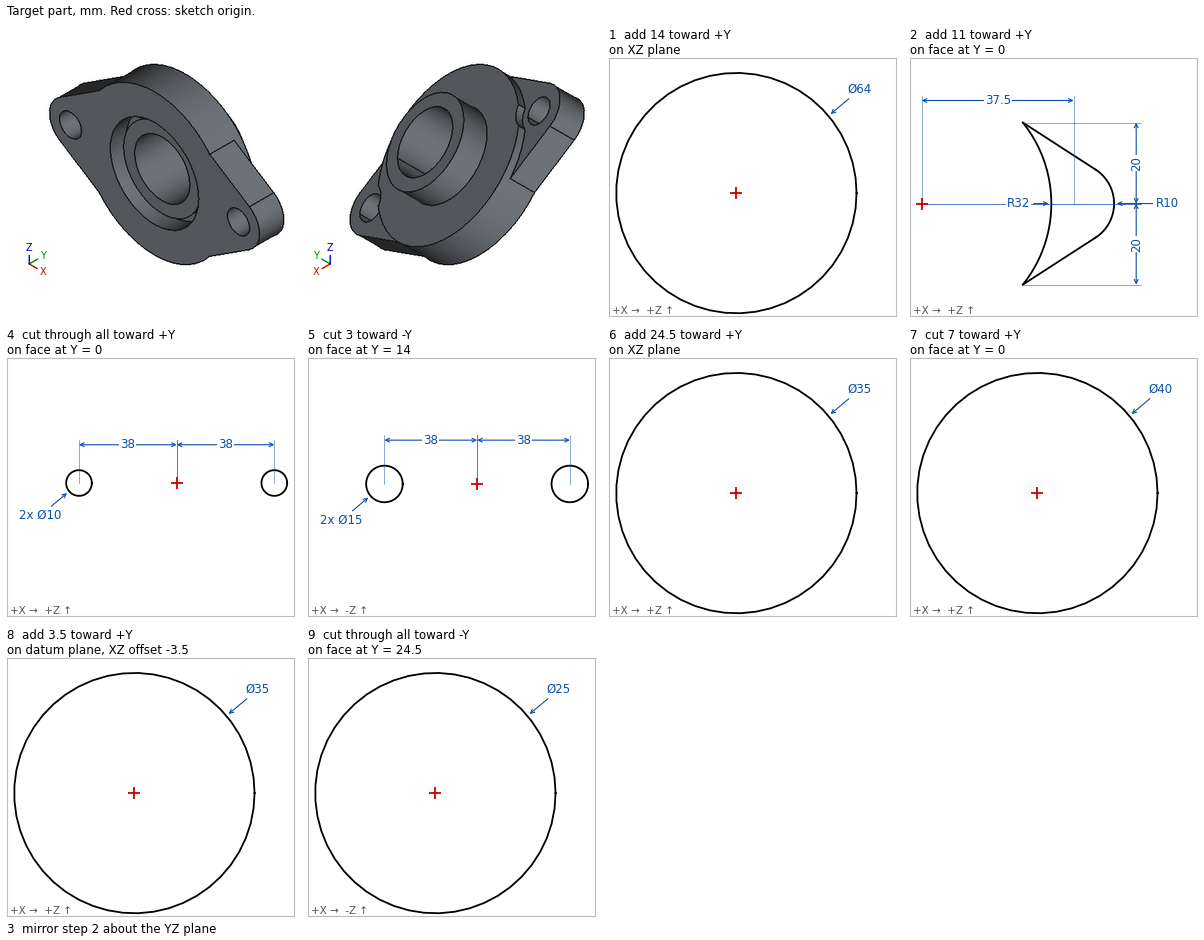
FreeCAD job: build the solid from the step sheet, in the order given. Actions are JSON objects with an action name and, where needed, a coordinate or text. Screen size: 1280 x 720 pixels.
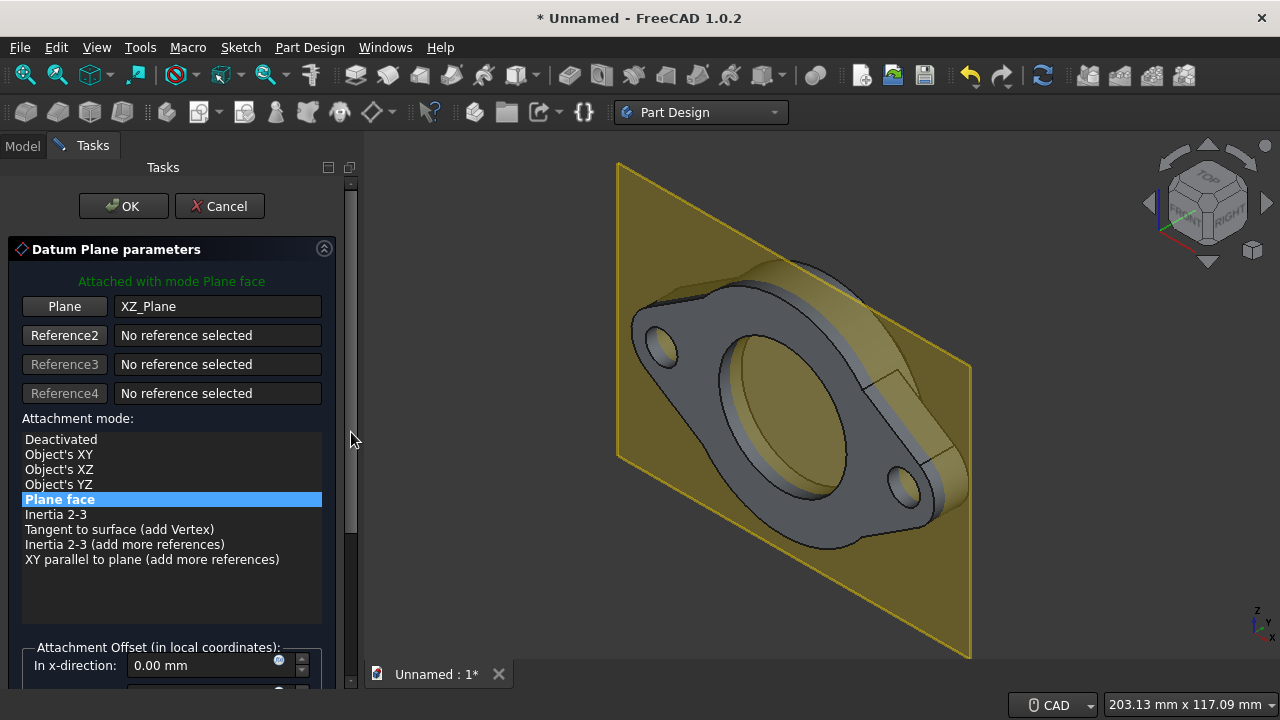
{"action": "left_click", "coordinate": [124, 206]}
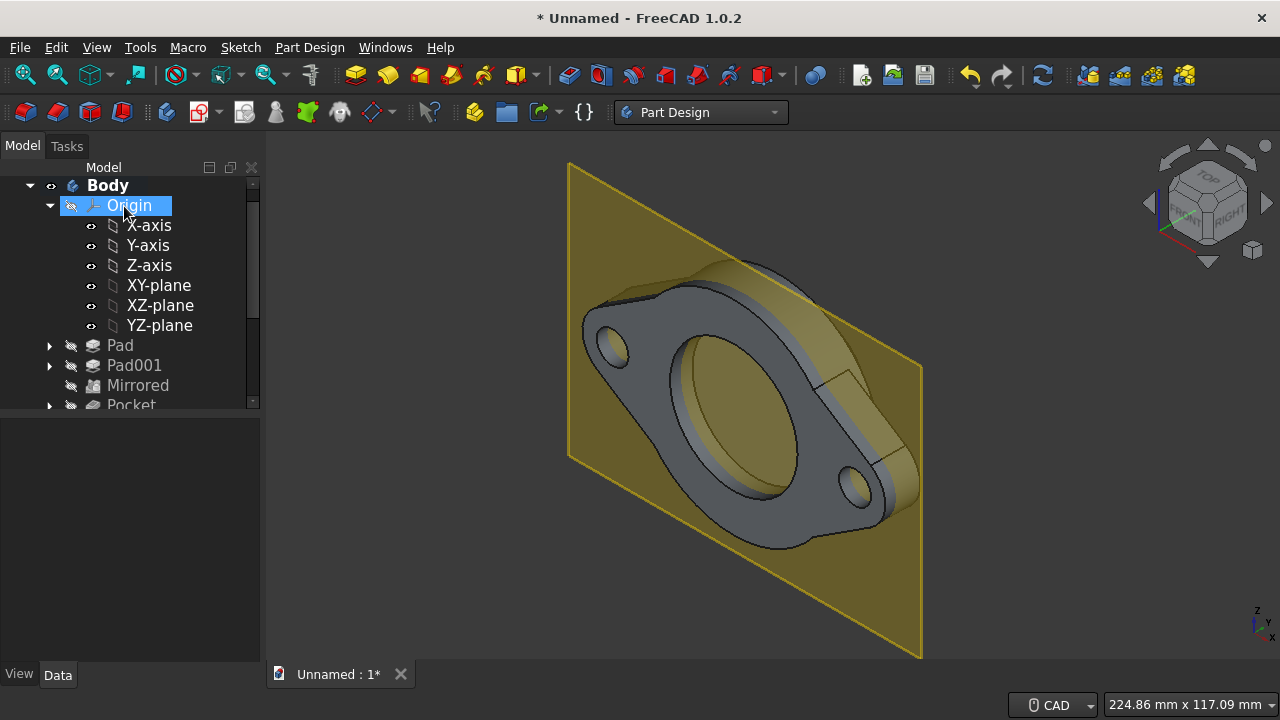
{"action": "scroll", "coordinate": [120, 301], "scroll_direction": "down", "scroll_amount": 3}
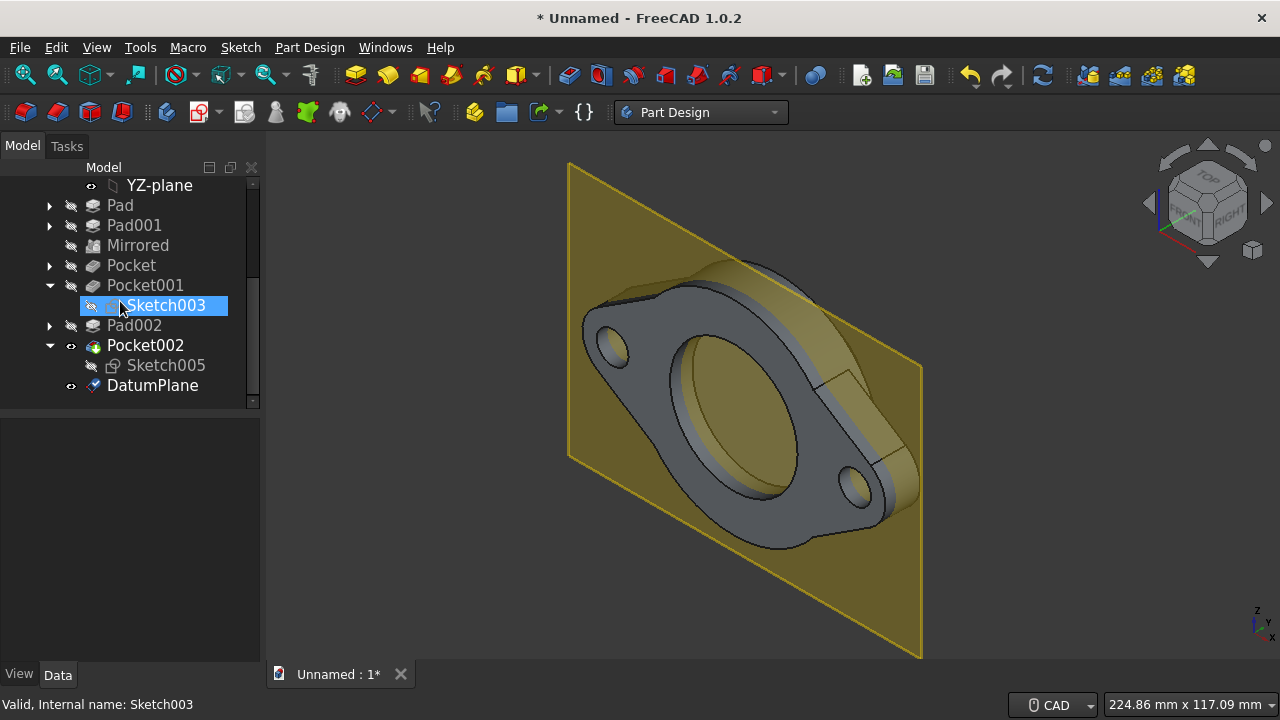
{"action": "left_click", "coordinate": [116, 386]}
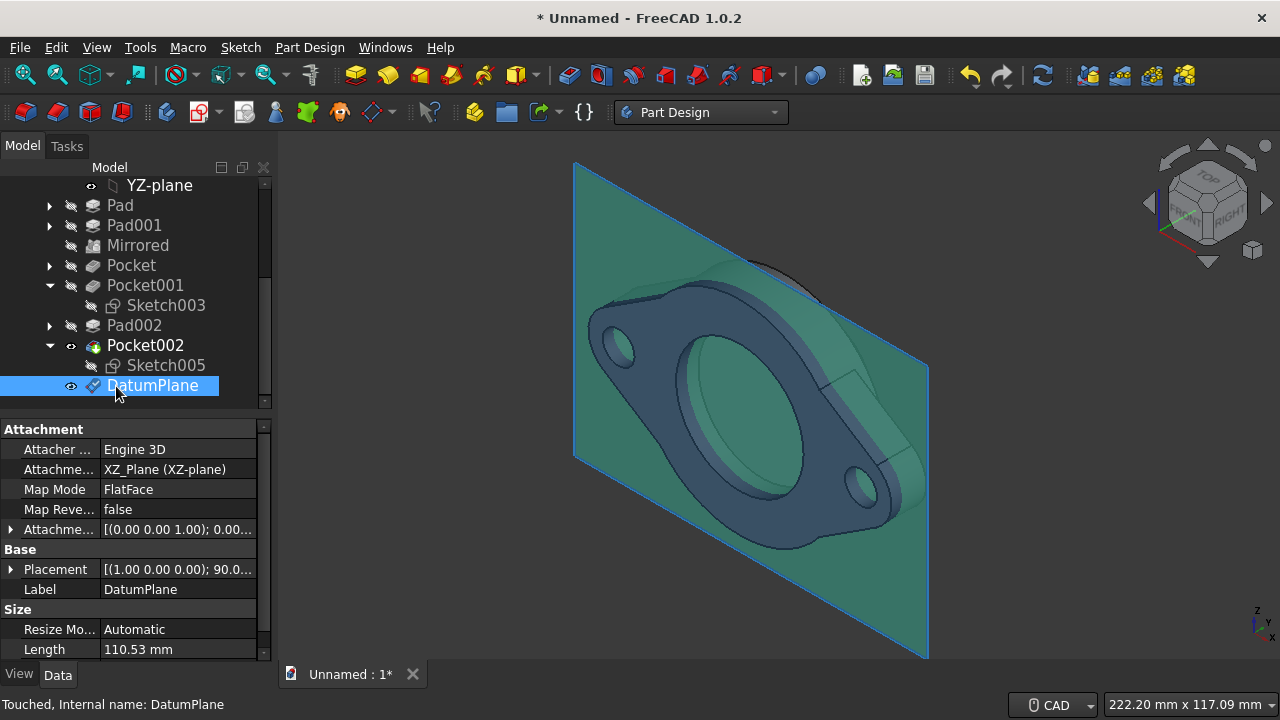
{"action": "left_click", "coordinate": [200, 112]}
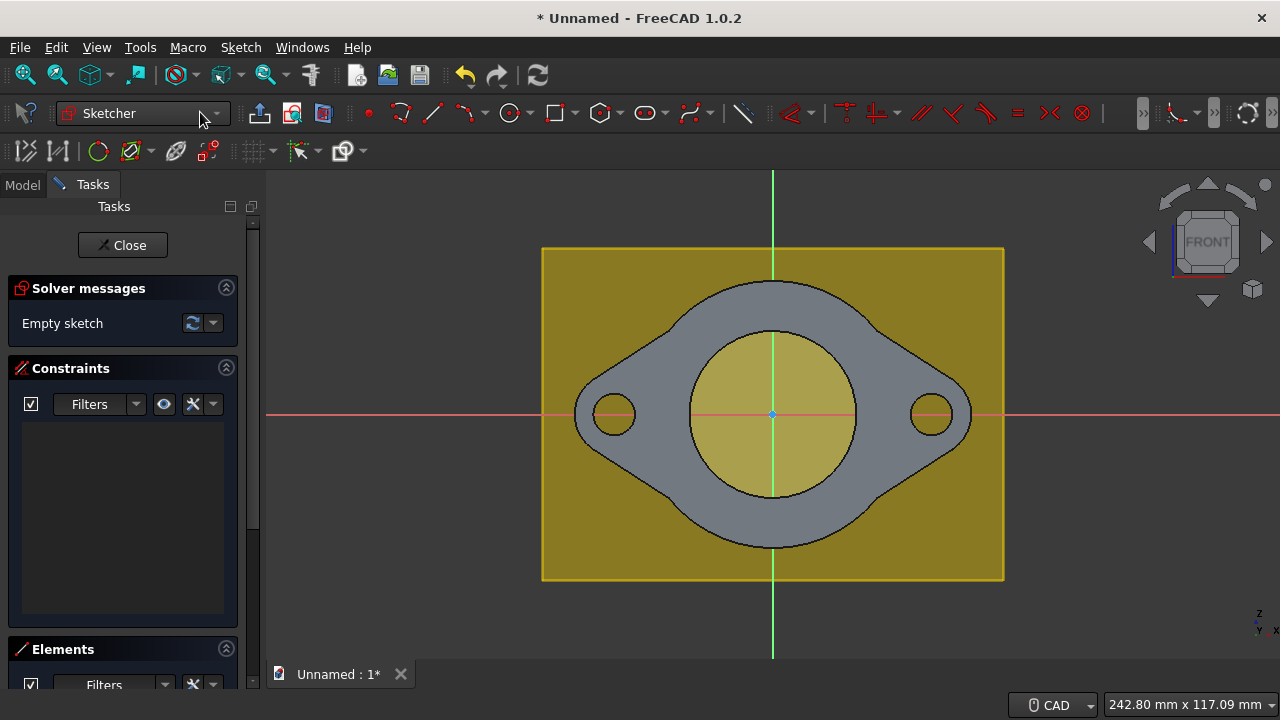
{"action": "left_click", "coordinate": [324, 114]}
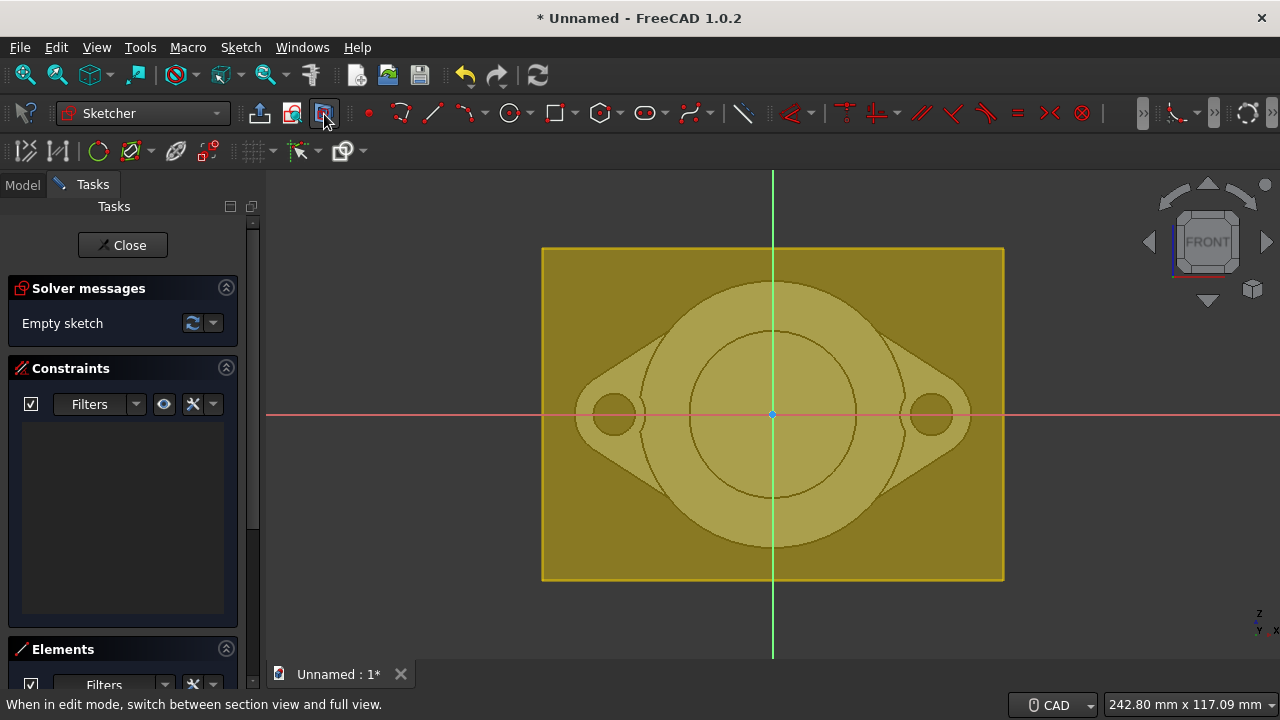
{"action": "scroll", "coordinate": [829, 415], "scroll_direction": "up", "scroll_amount": 4}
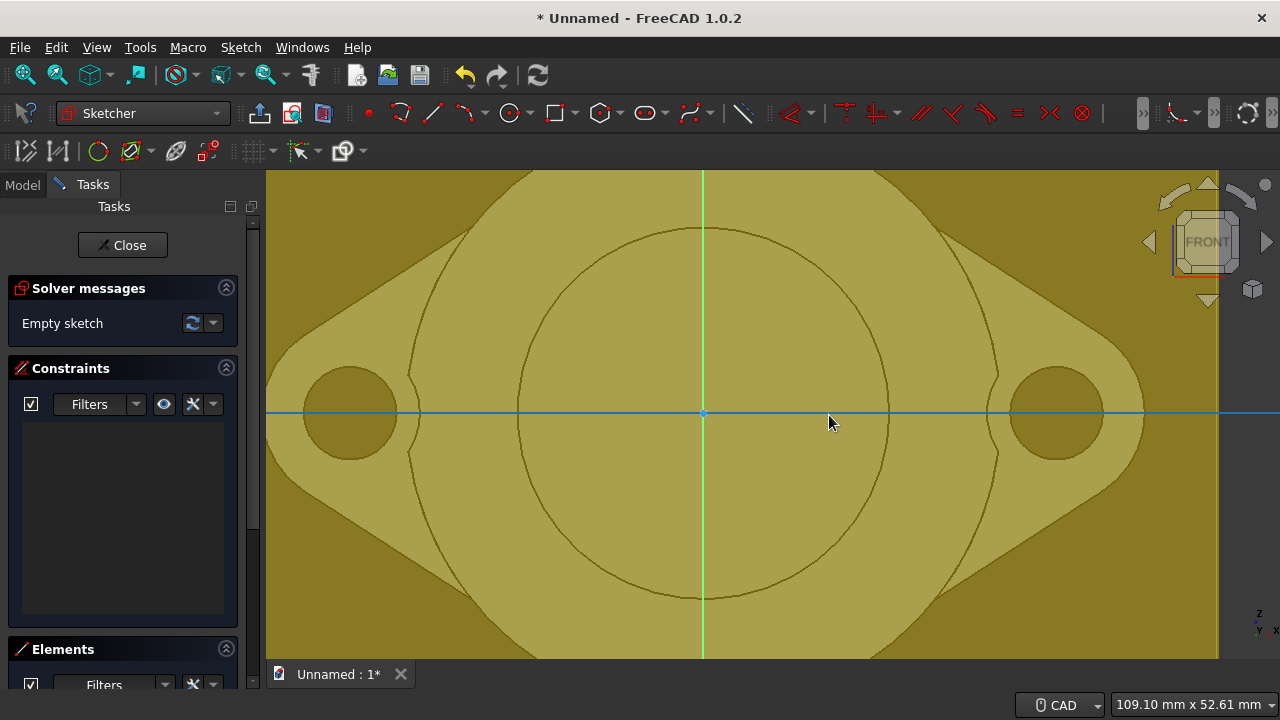
{"action": "left_click", "coordinate": [510, 114]}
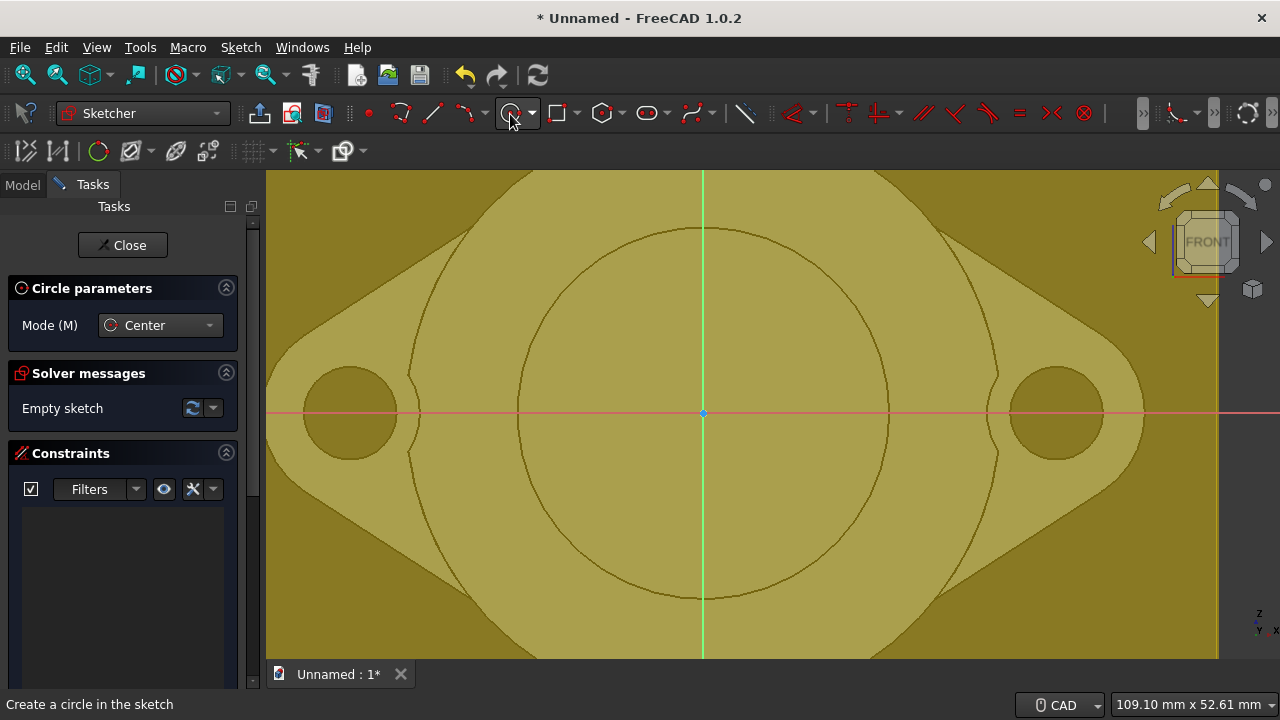
{"action": "left_click", "coordinate": [703, 413]}
{"action": "left_click", "coordinate": [818, 298]}
{"action": "key", "text": "Escape"}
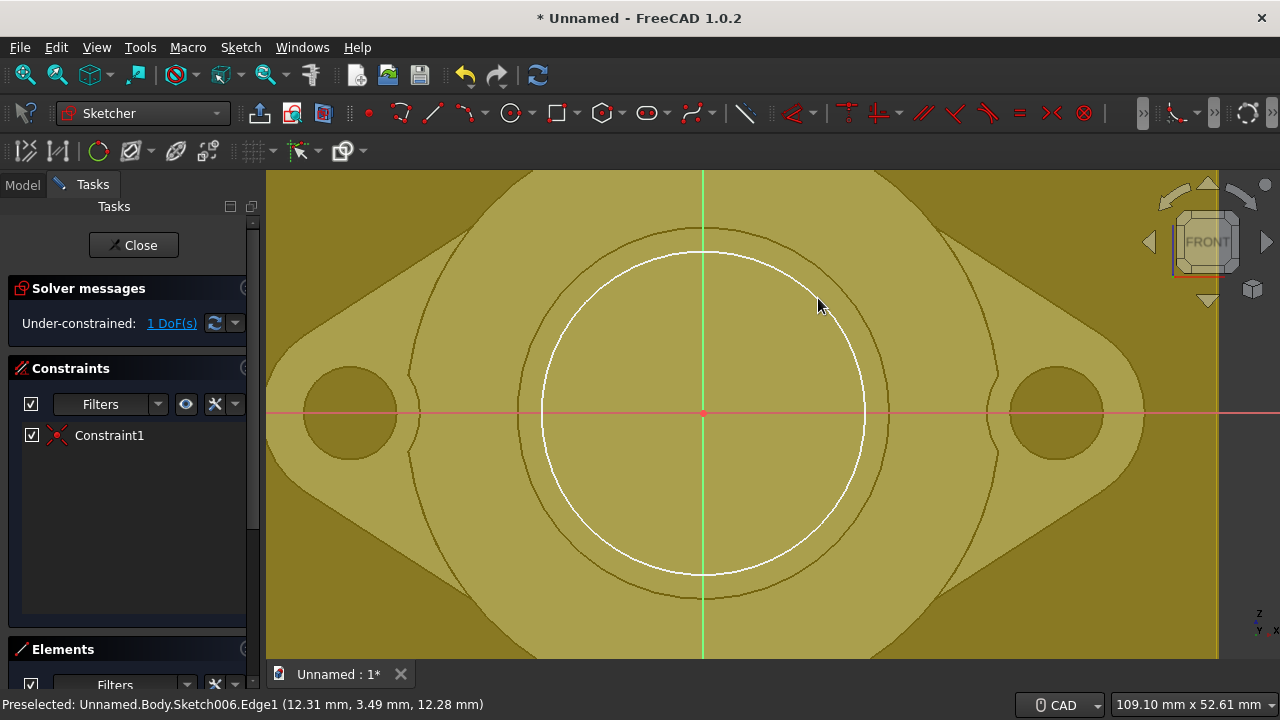
{"action": "key", "text": "d"}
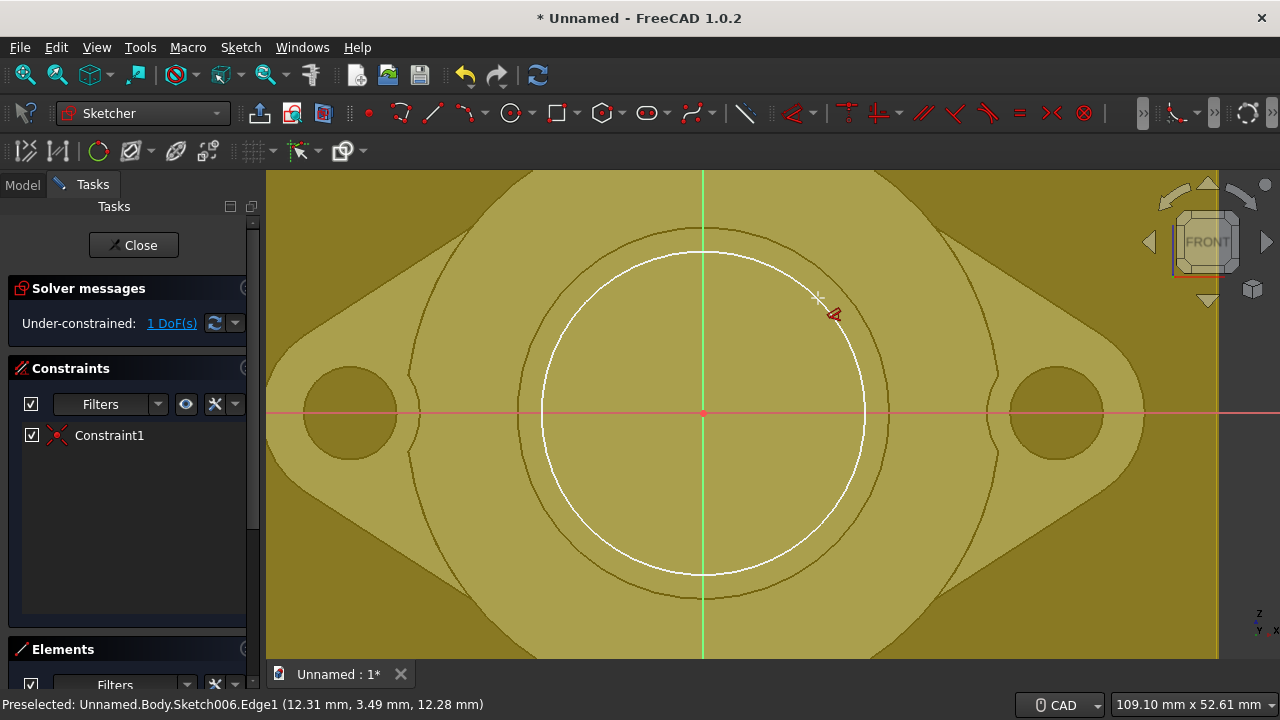
{"action": "left_click", "coordinate": [817, 298]}
{"action": "left_click", "coordinate": [839, 275]}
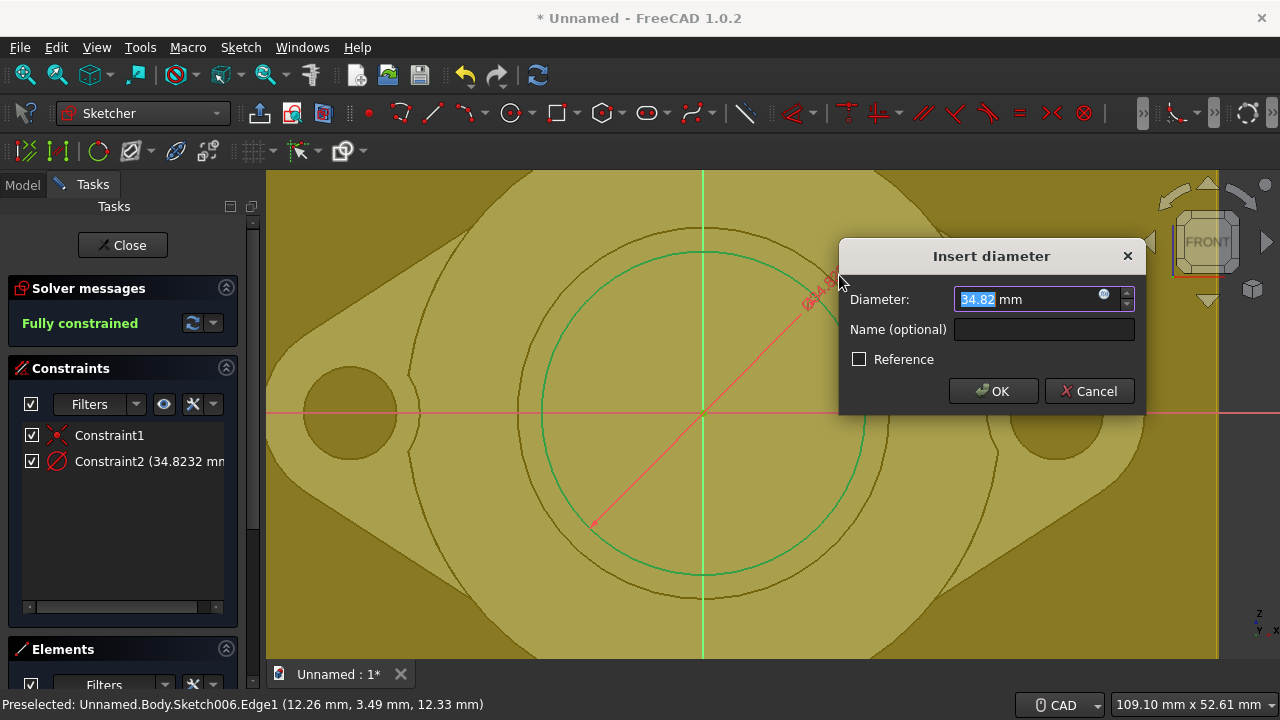
{"action": "type", "text": "35"}
{"action": "key", "text": "Return"}
{"action": "key", "text": "Escape"}